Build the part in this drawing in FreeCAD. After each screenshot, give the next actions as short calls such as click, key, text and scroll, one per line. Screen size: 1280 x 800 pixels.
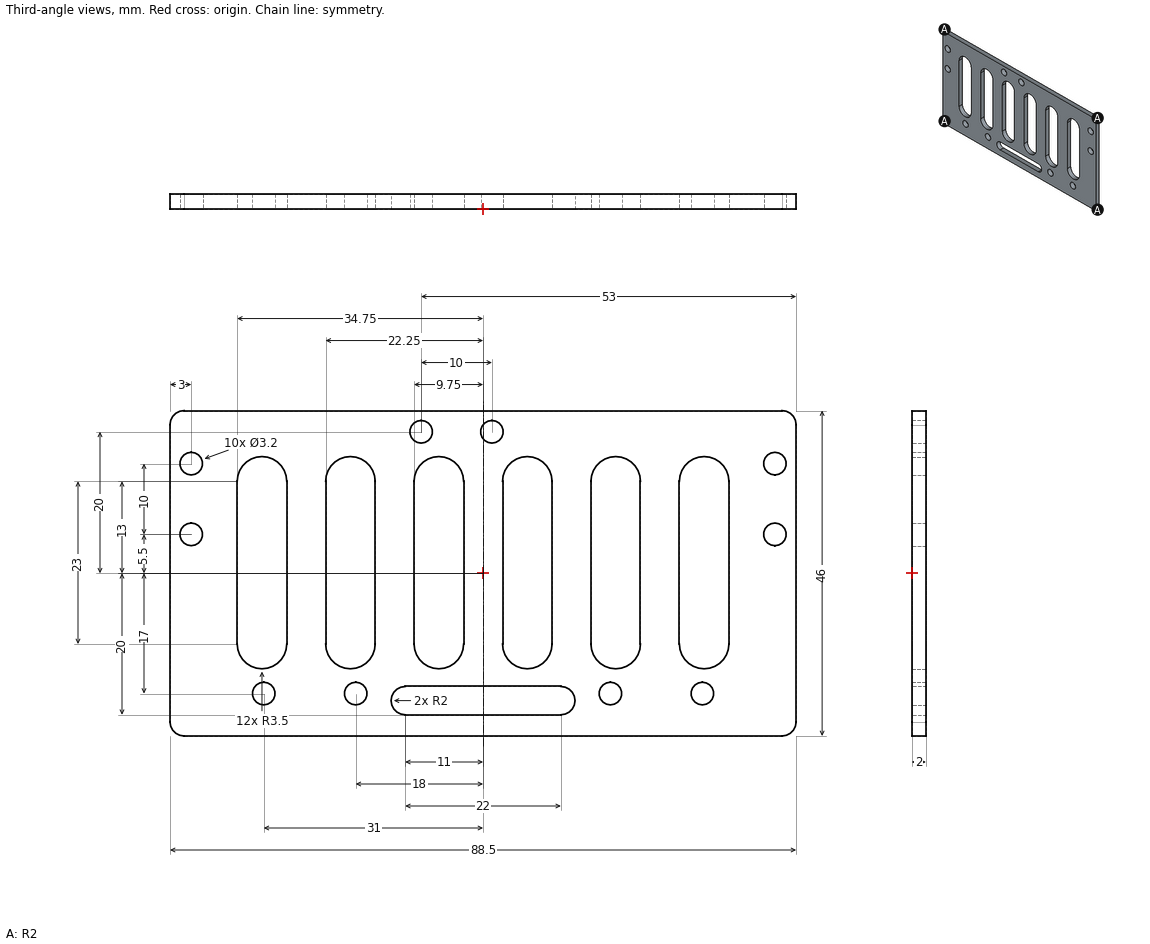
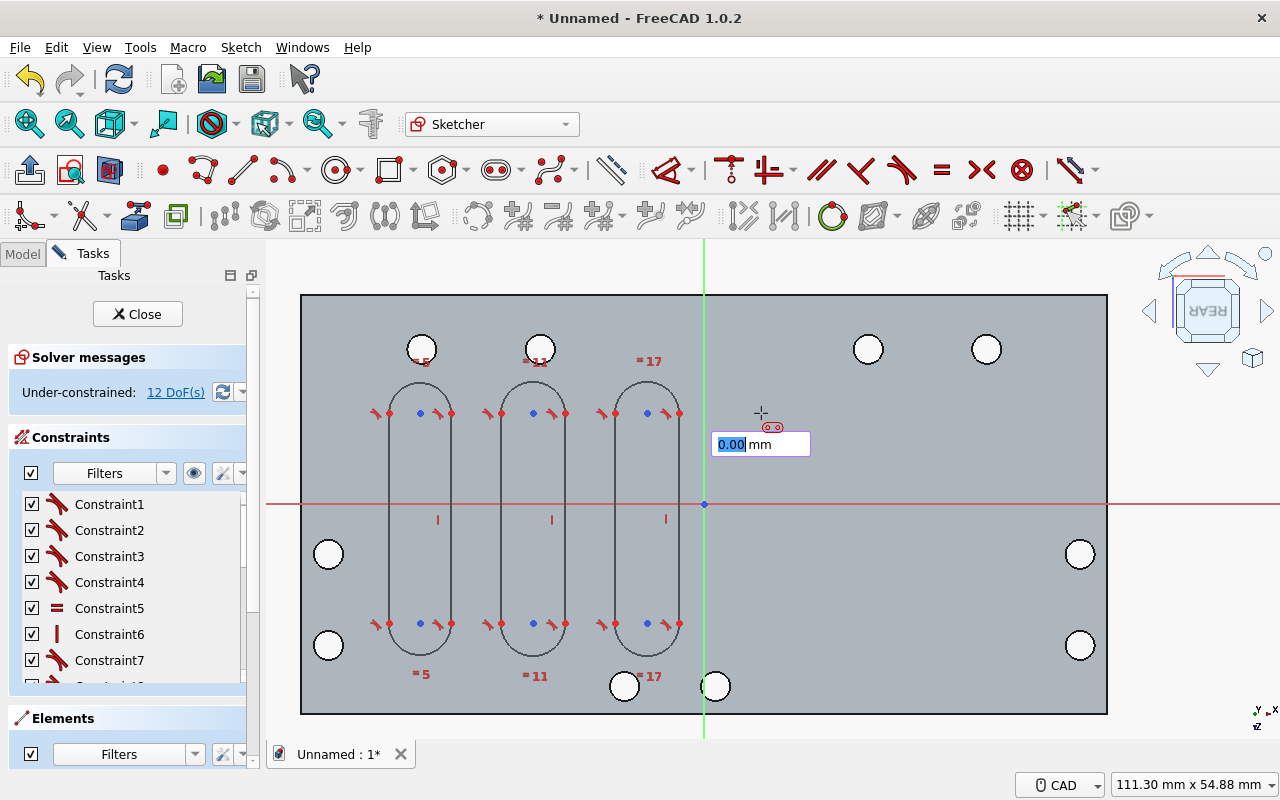
click(793, 549)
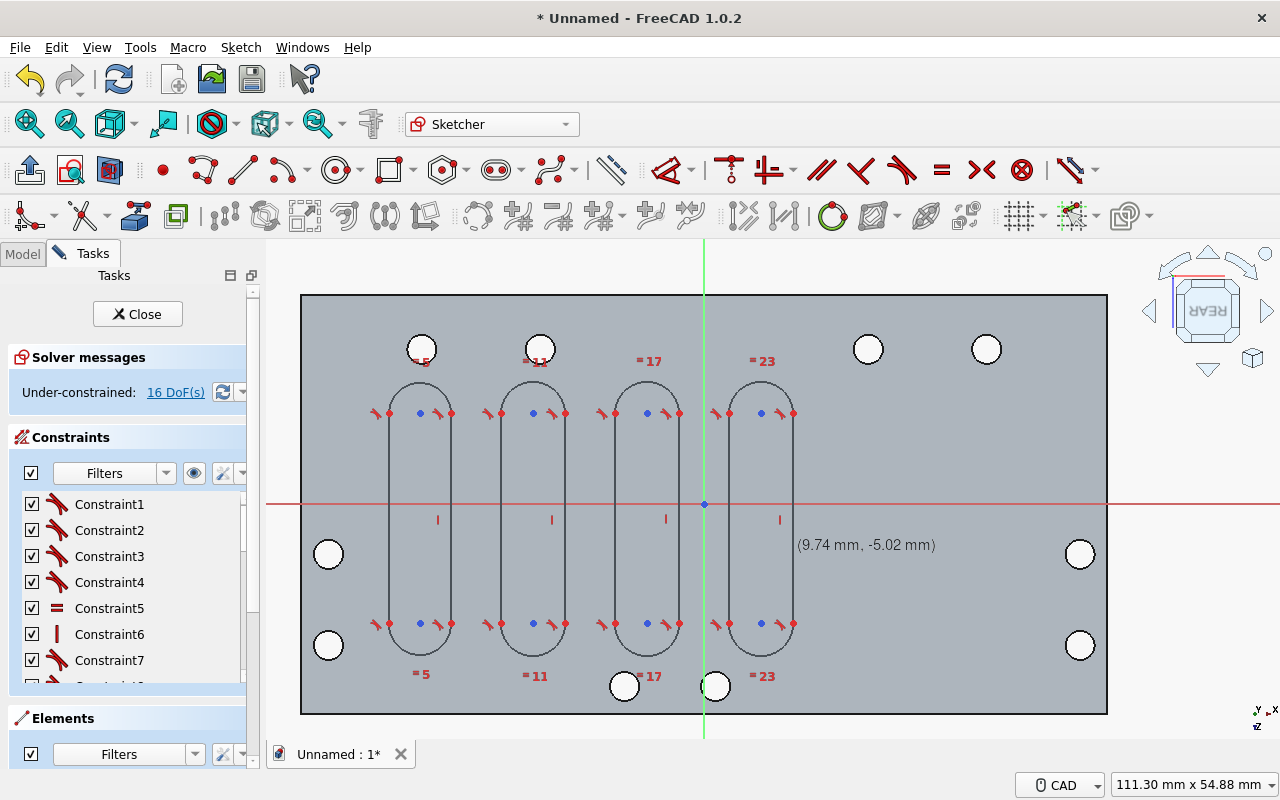
click(875, 623)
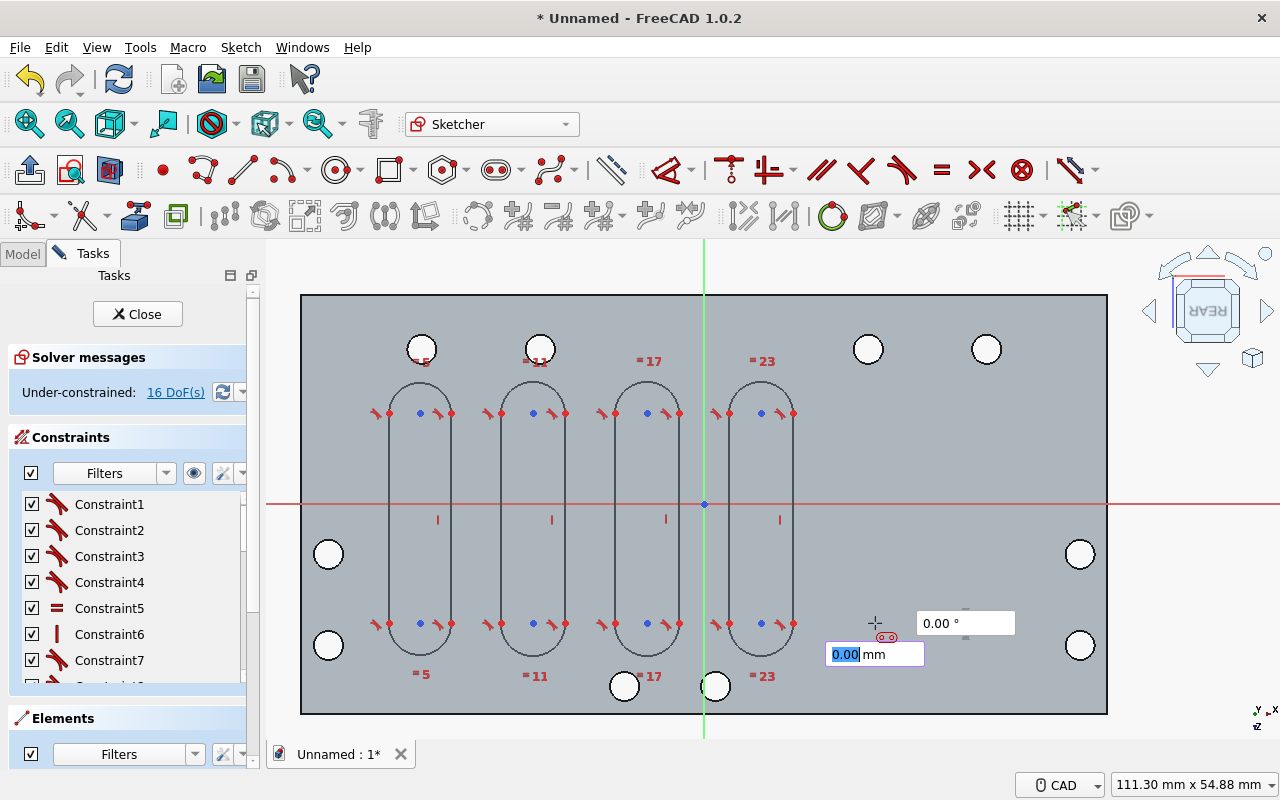
click(875, 413)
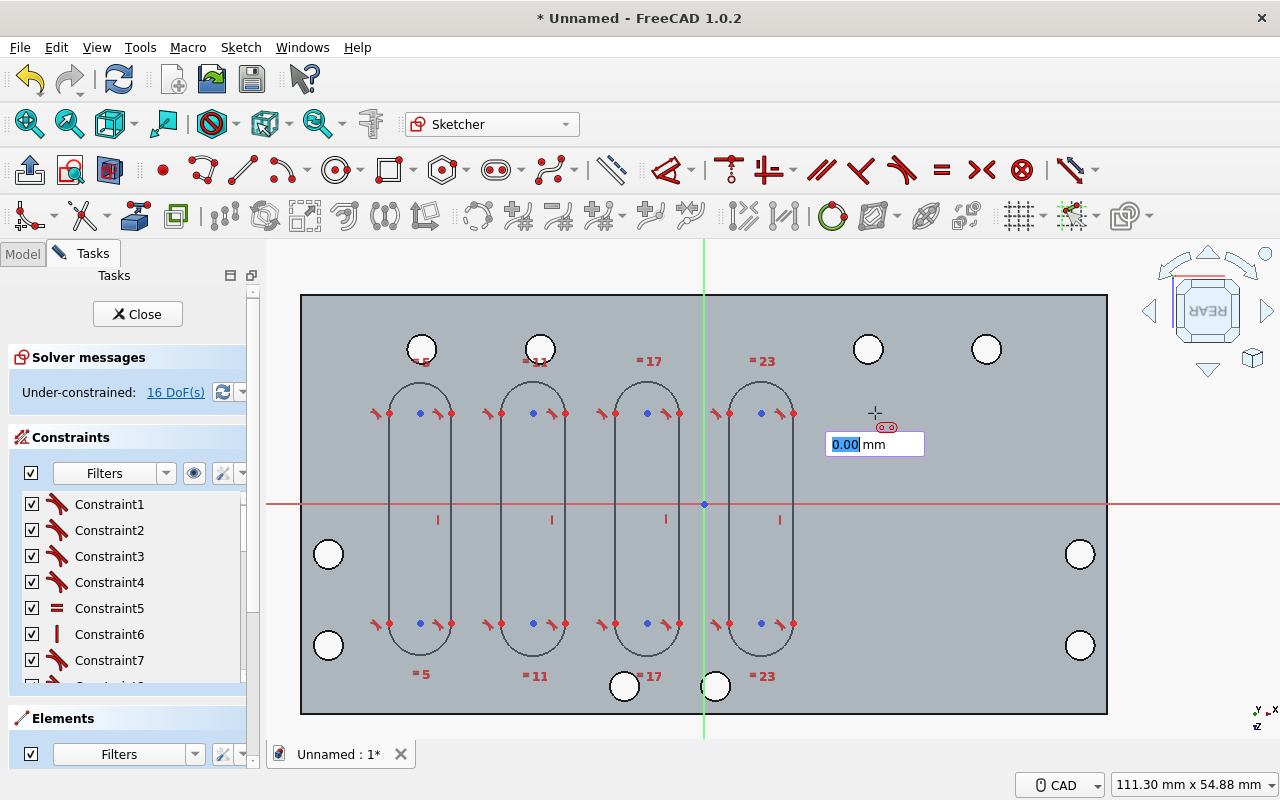
click(907, 549)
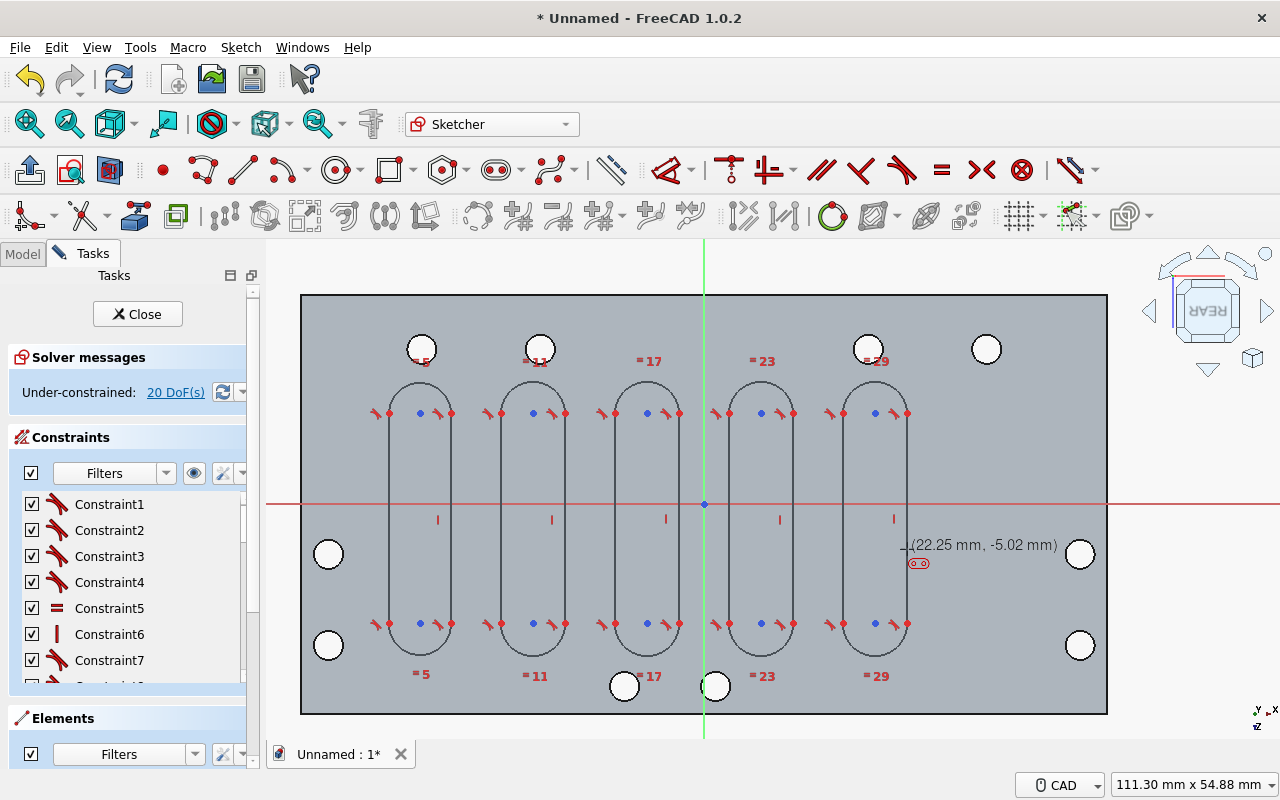
click(989, 623)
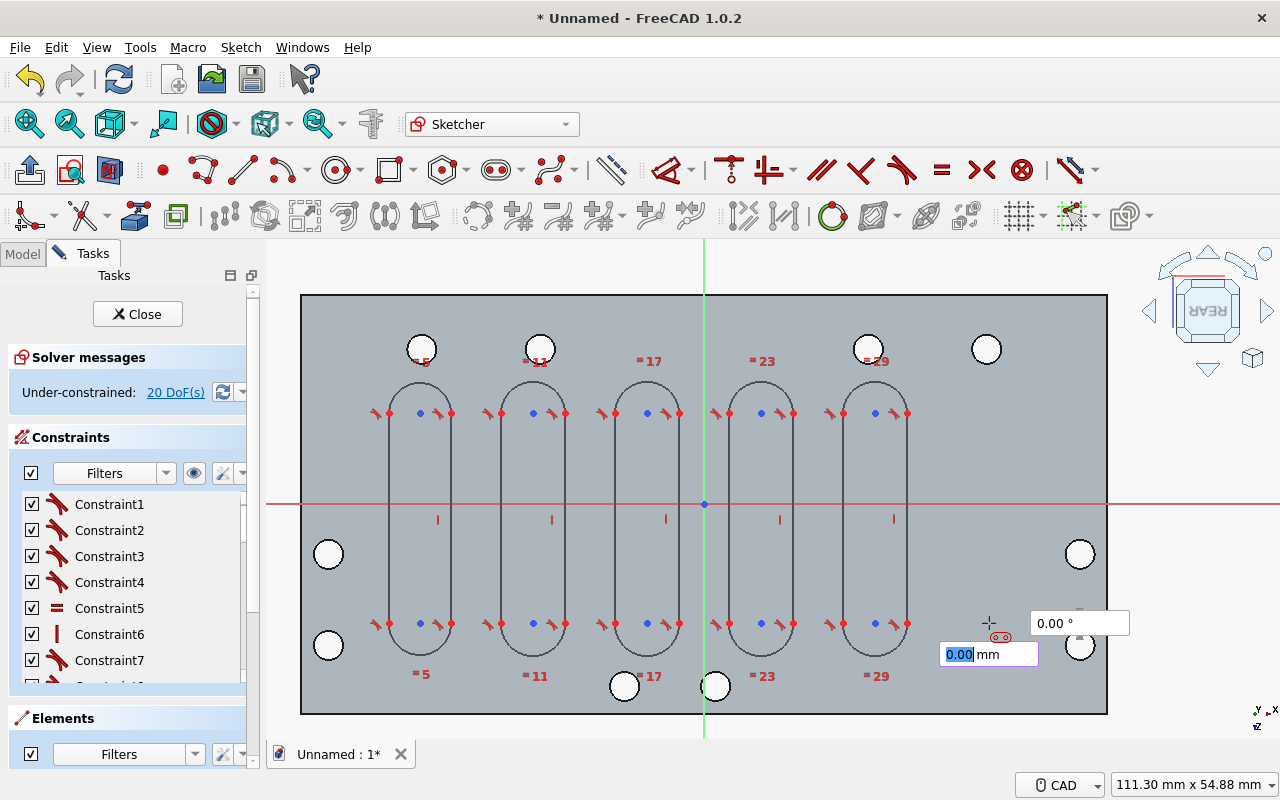
click(989, 413)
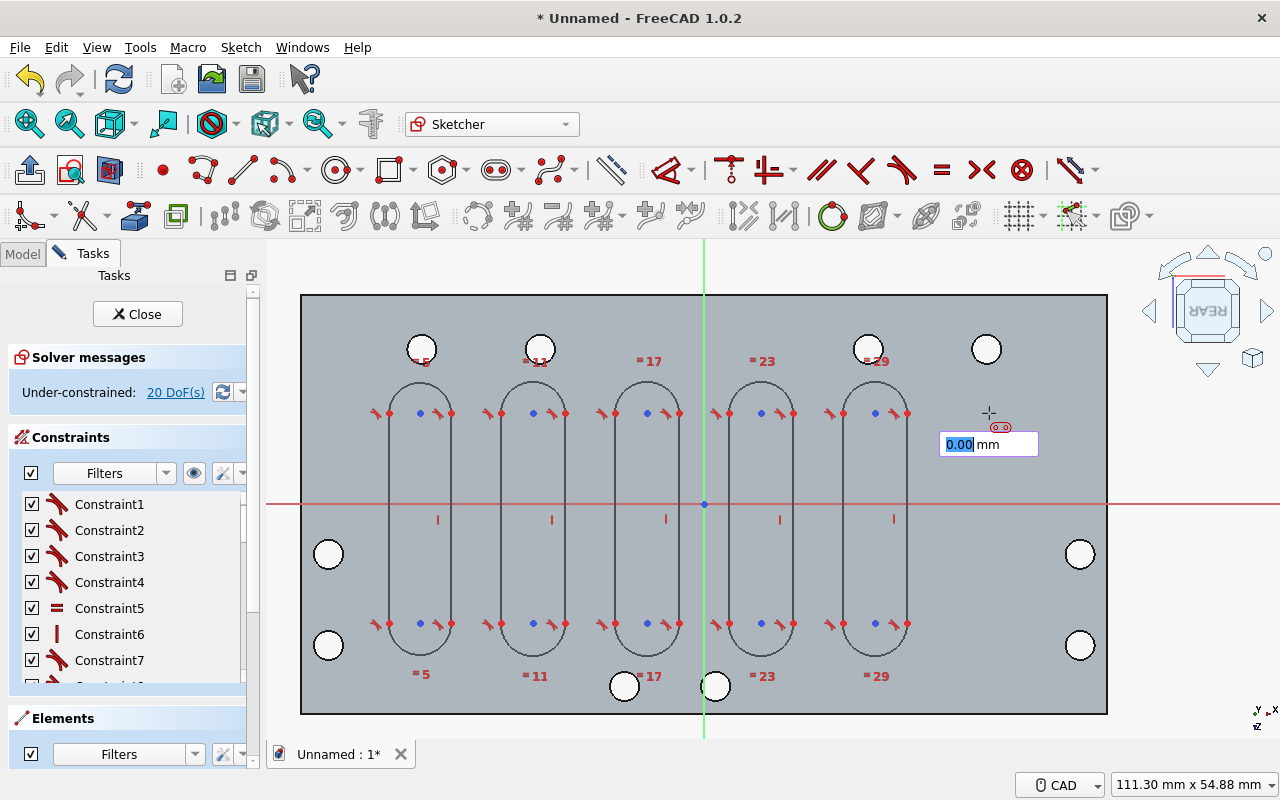
click(1021, 549)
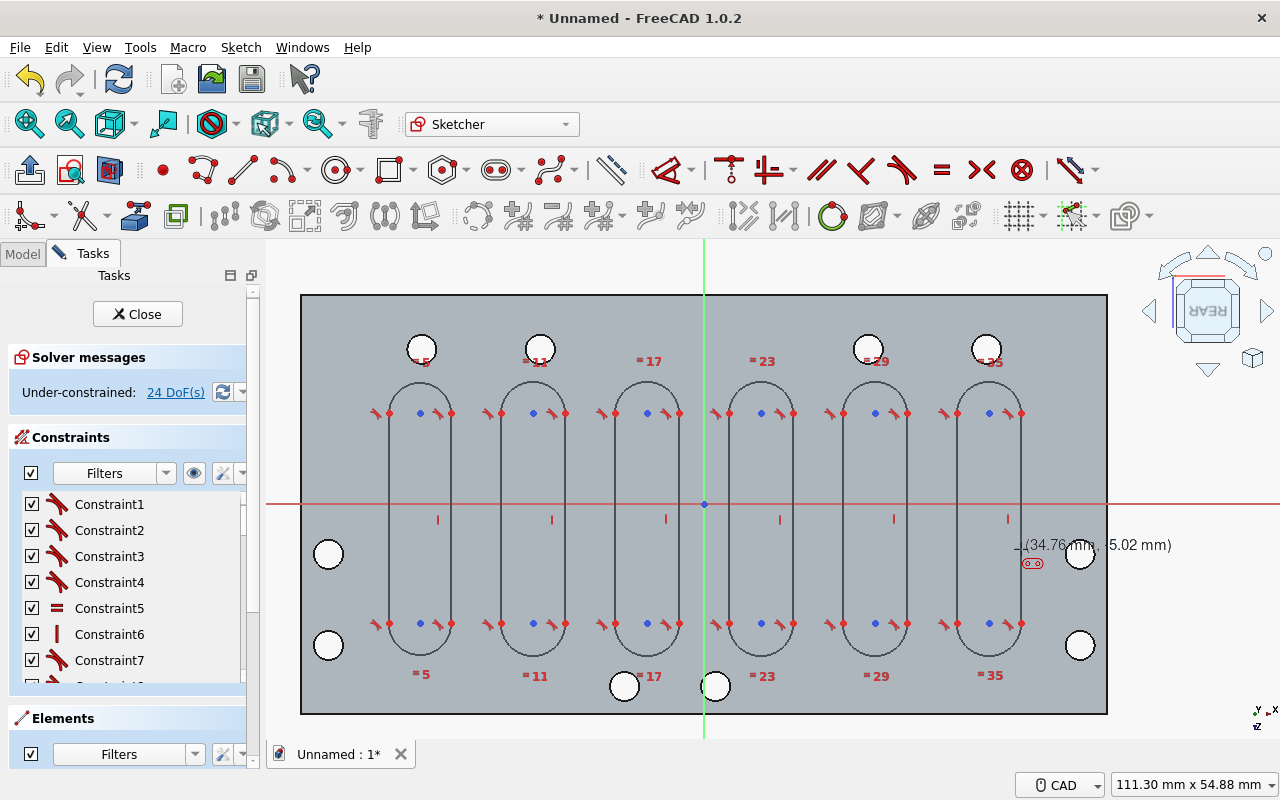
scroll(604, 340, up, 2)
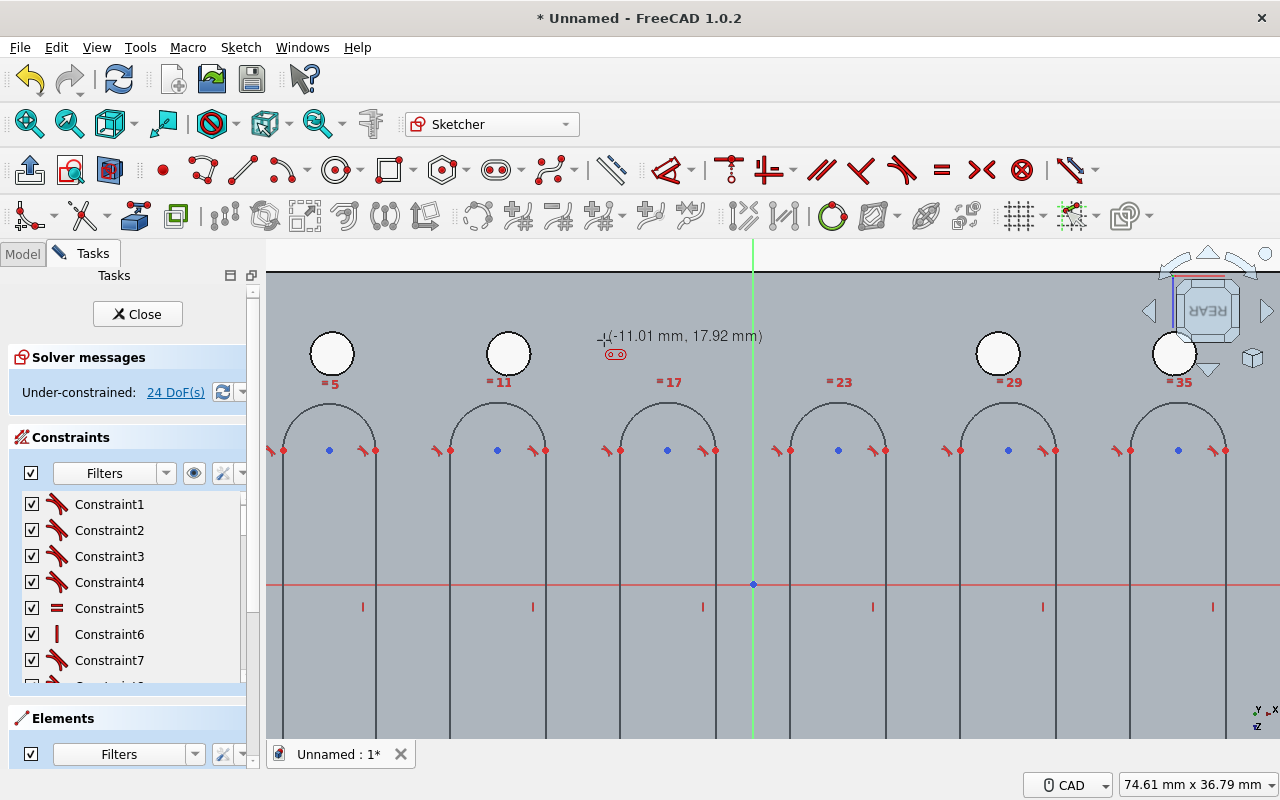
click(604, 340)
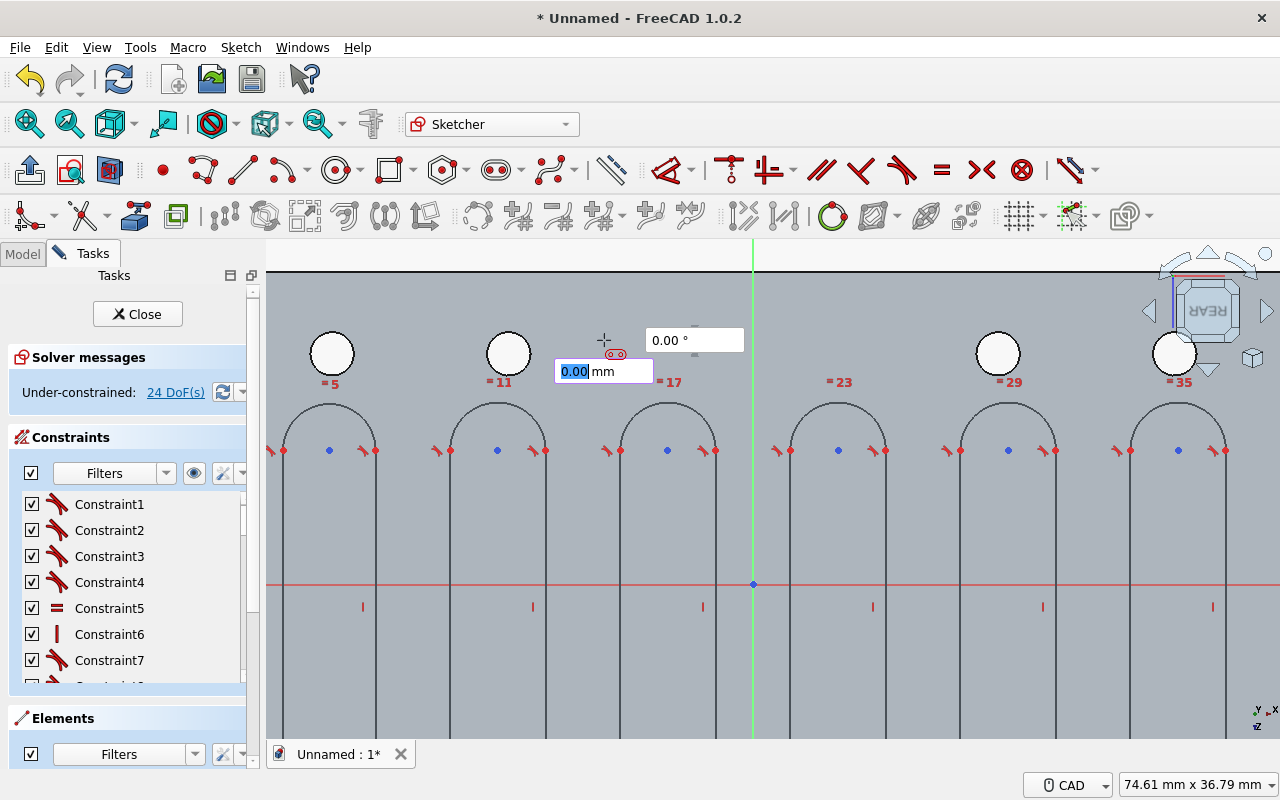
click(903, 340)